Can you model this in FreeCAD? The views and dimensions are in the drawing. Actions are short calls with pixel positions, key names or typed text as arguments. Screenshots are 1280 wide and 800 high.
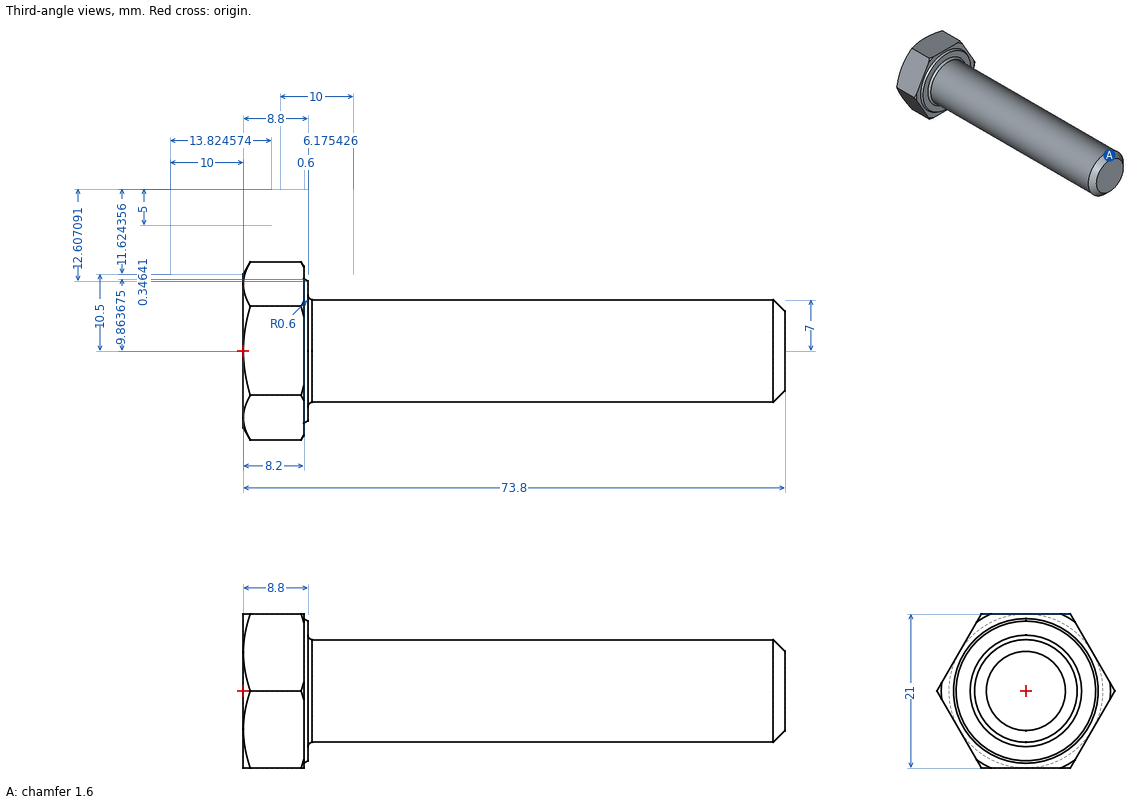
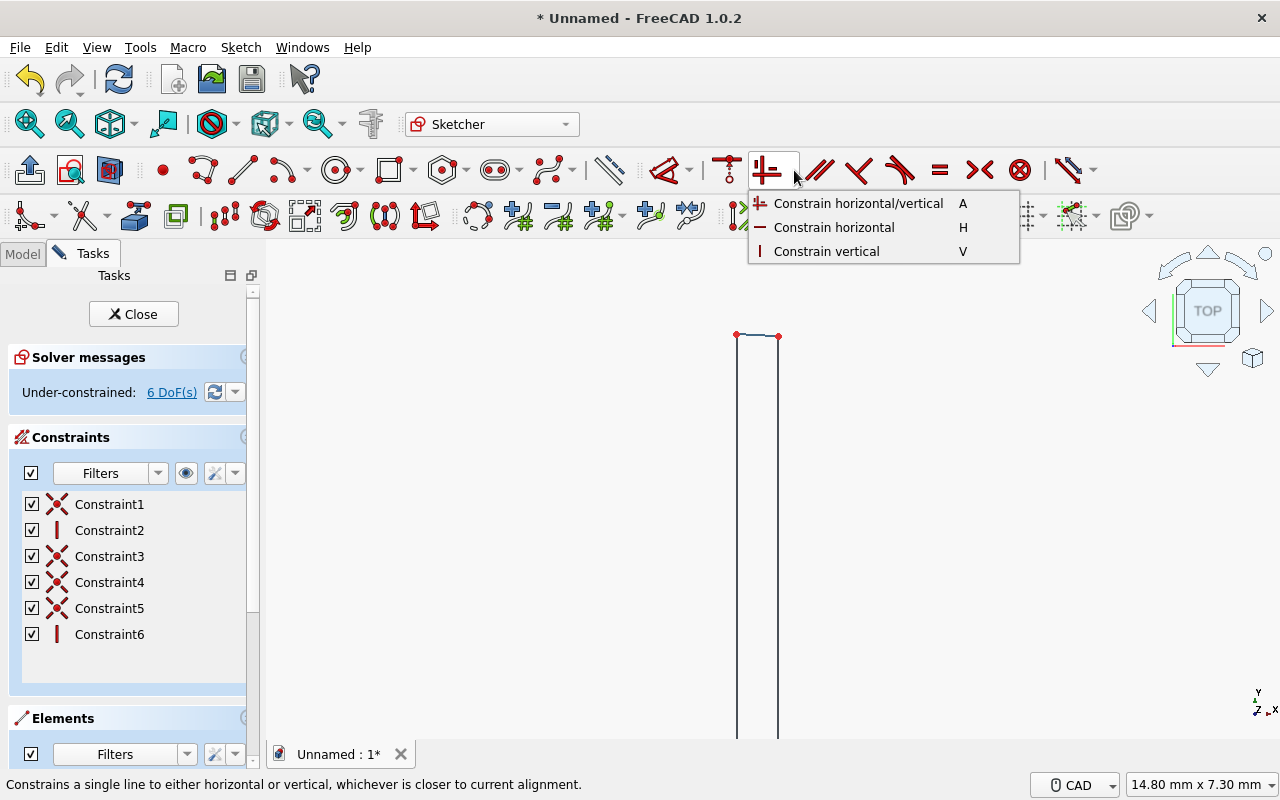
click(884, 227)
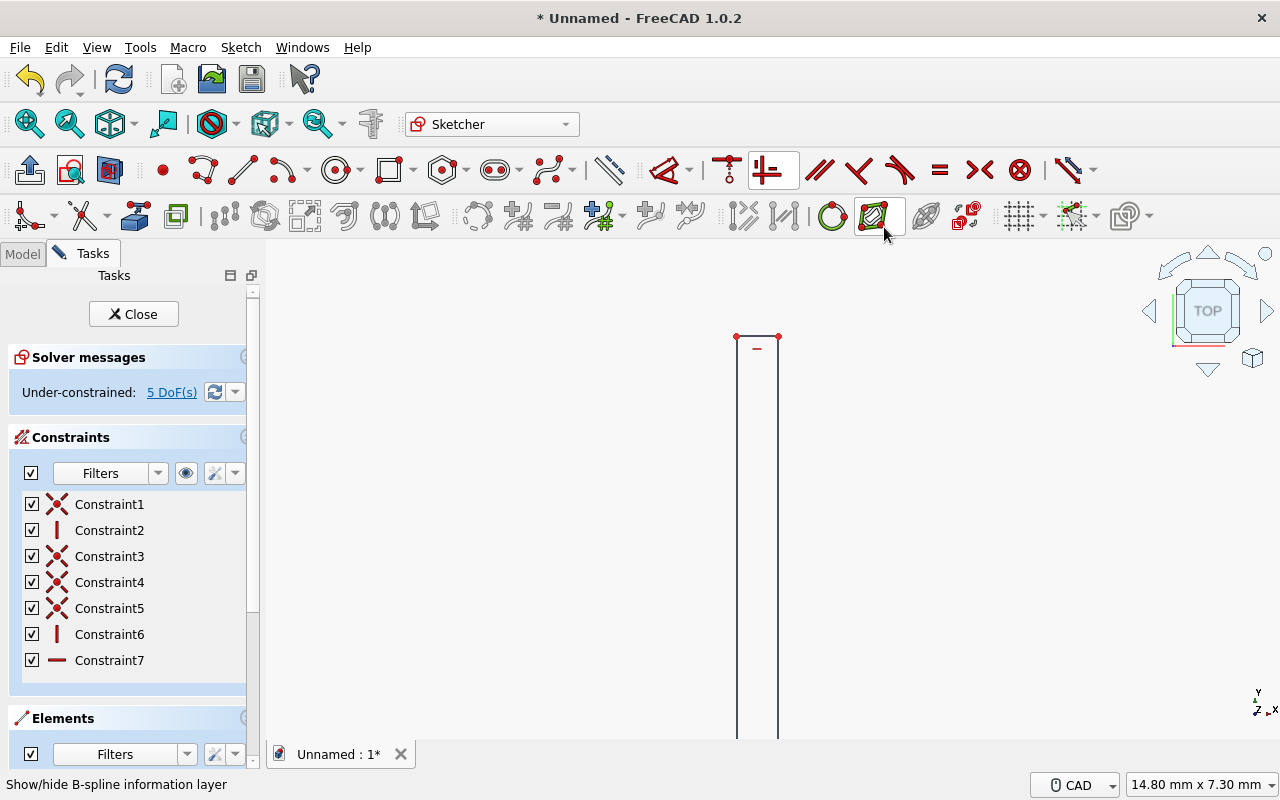
click(664, 170)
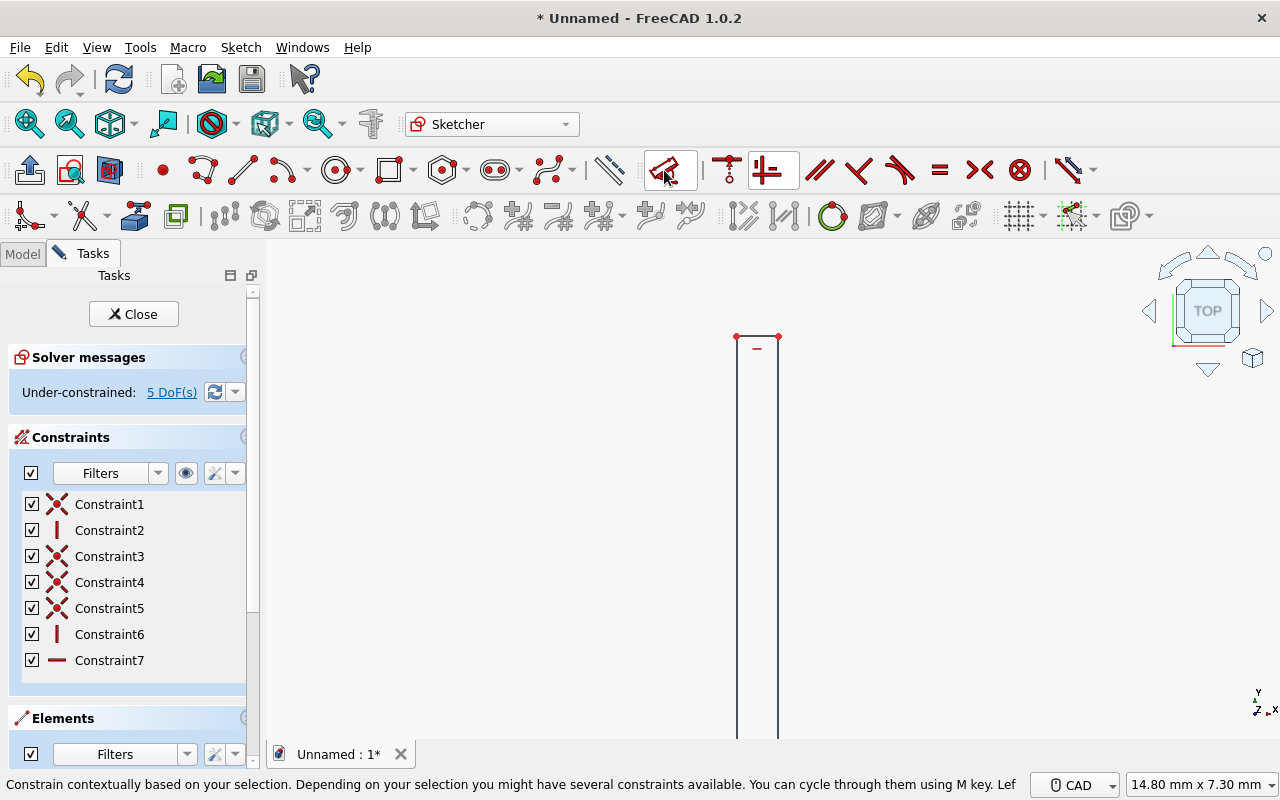
click(766, 336)
click(757, 302)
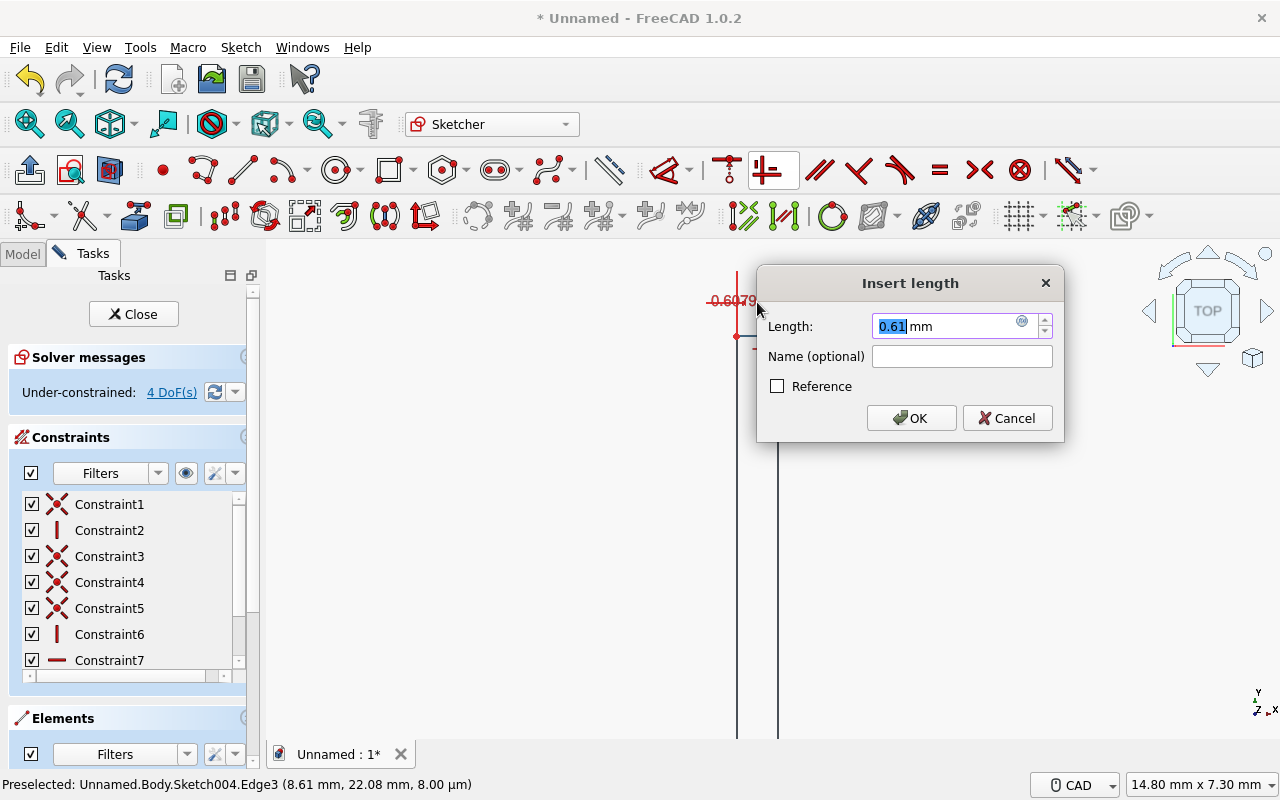
text(0.6)
key(Return)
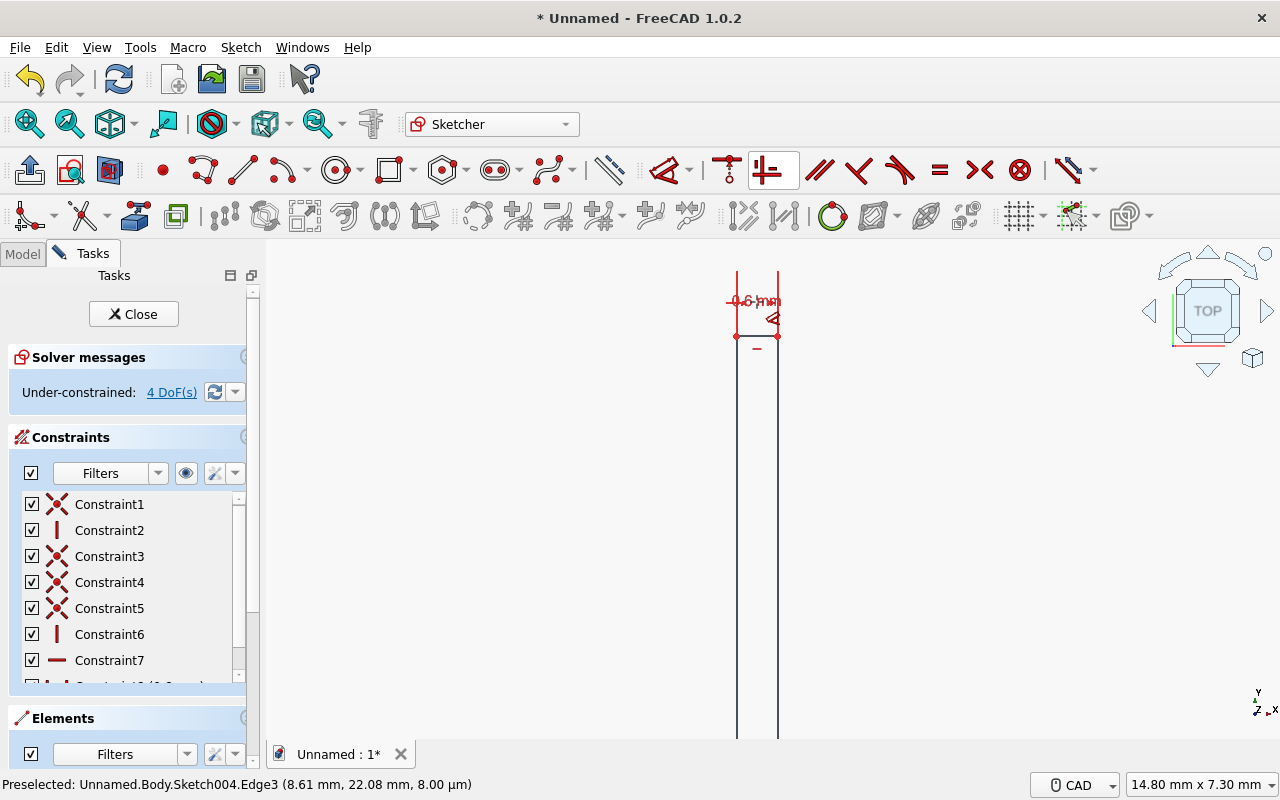
scroll(762, 337, down, 8)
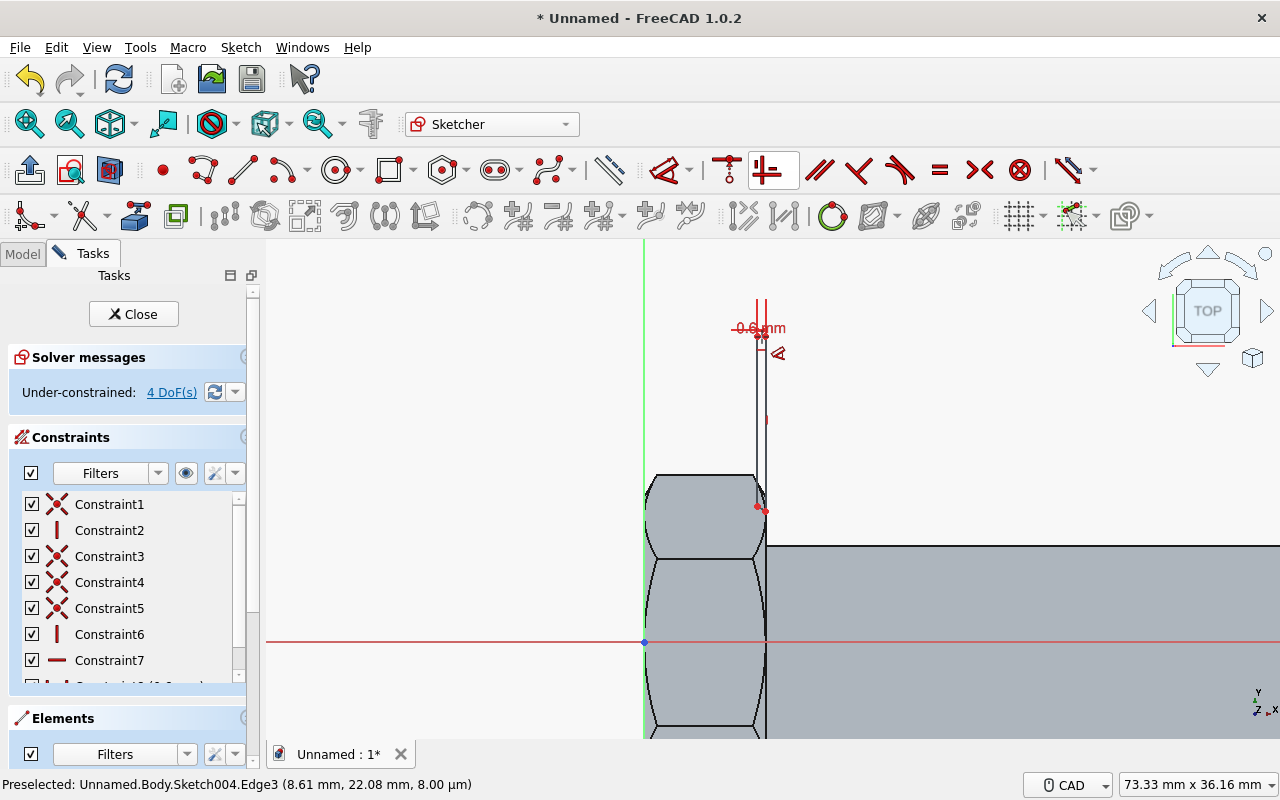
scroll(757, 506, up, 2)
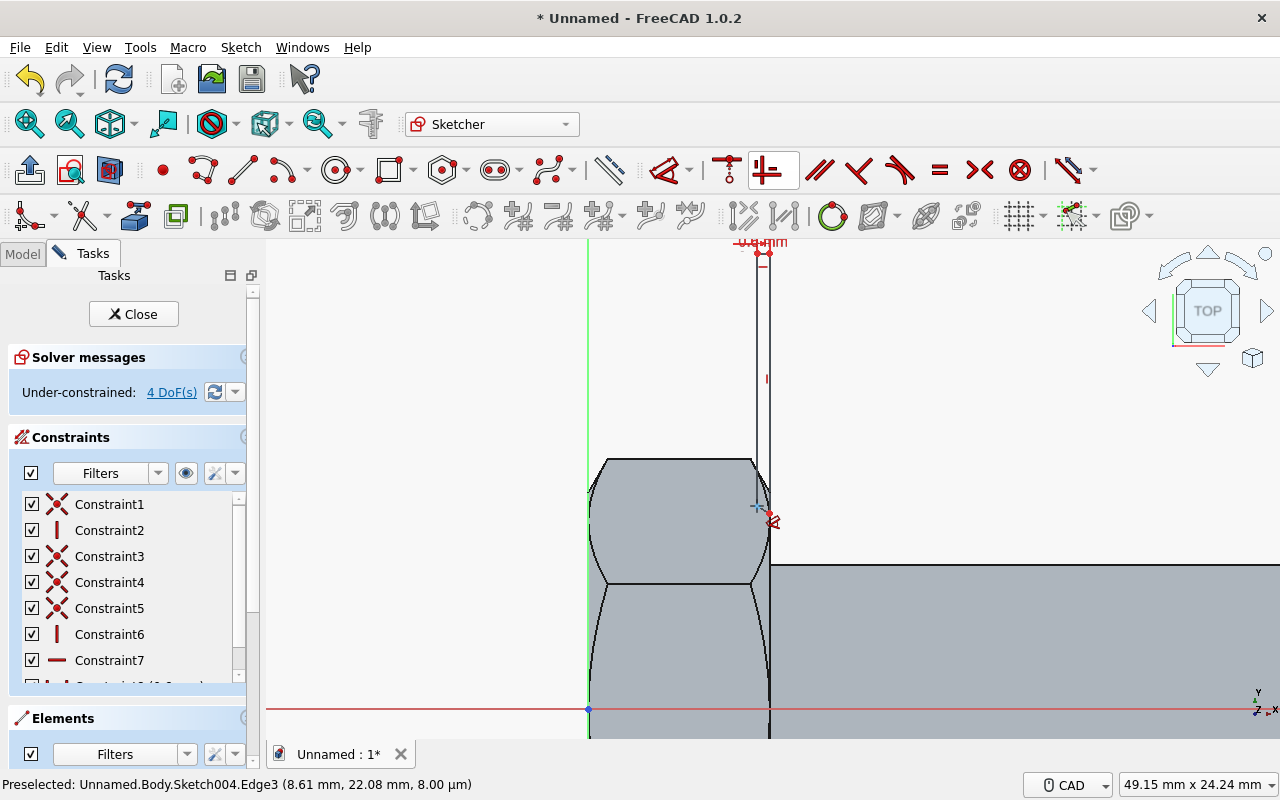
click(757, 506)
click(673, 472)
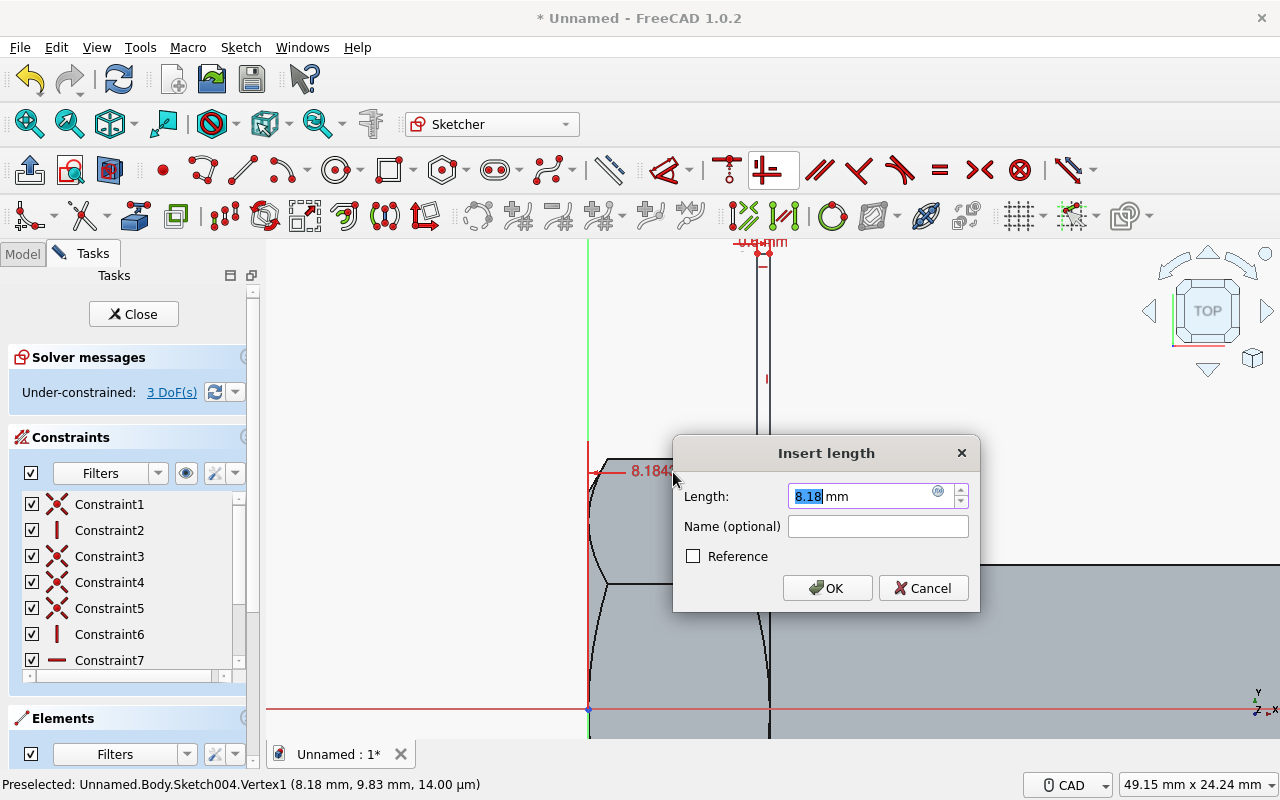
text(8.2)
key(Return)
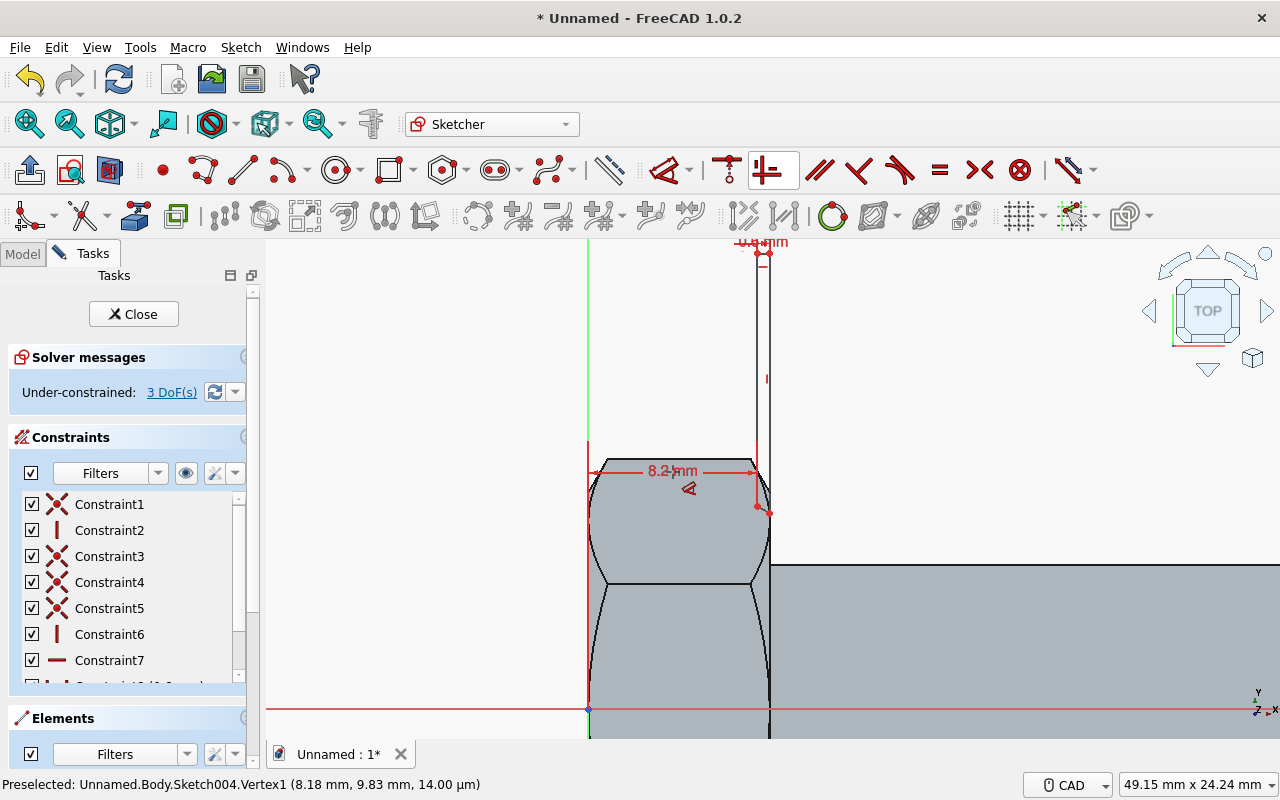
scroll(764, 510, up, 9)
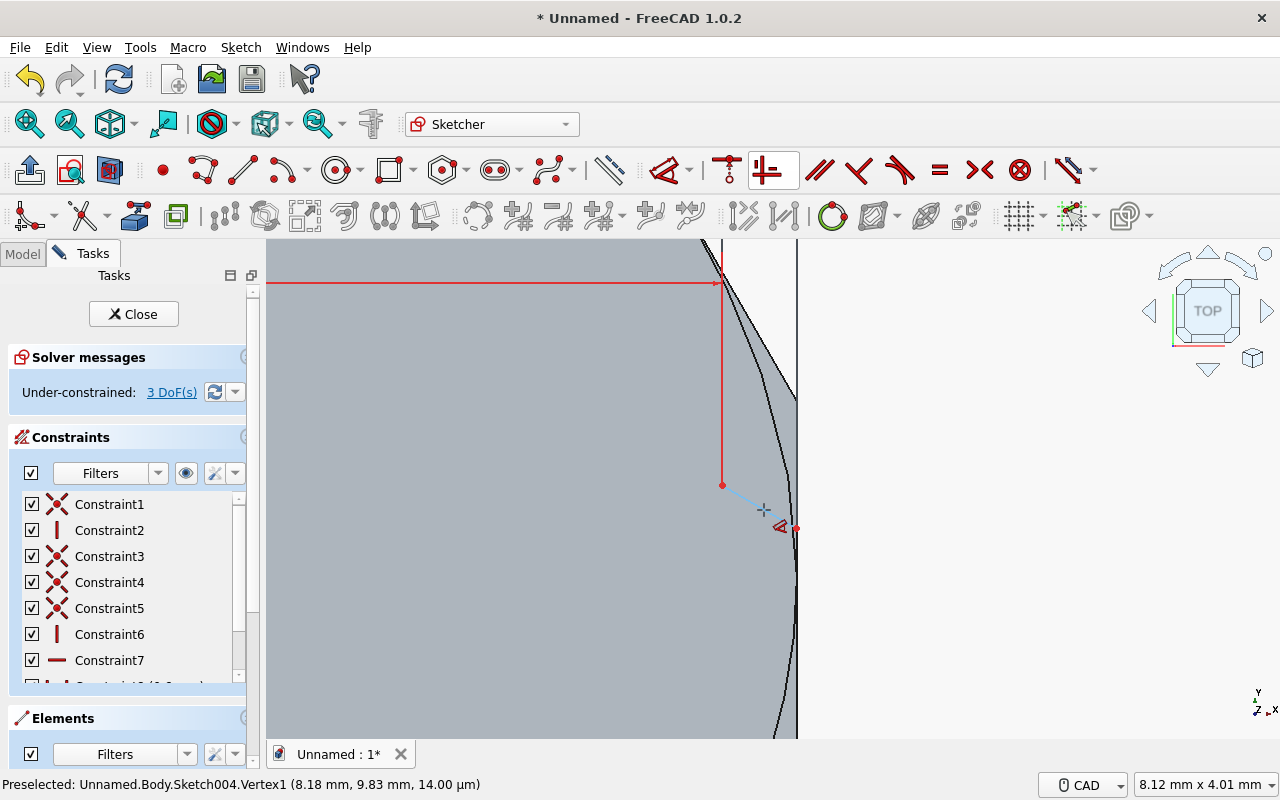
click(760, 507)
click(831, 507)